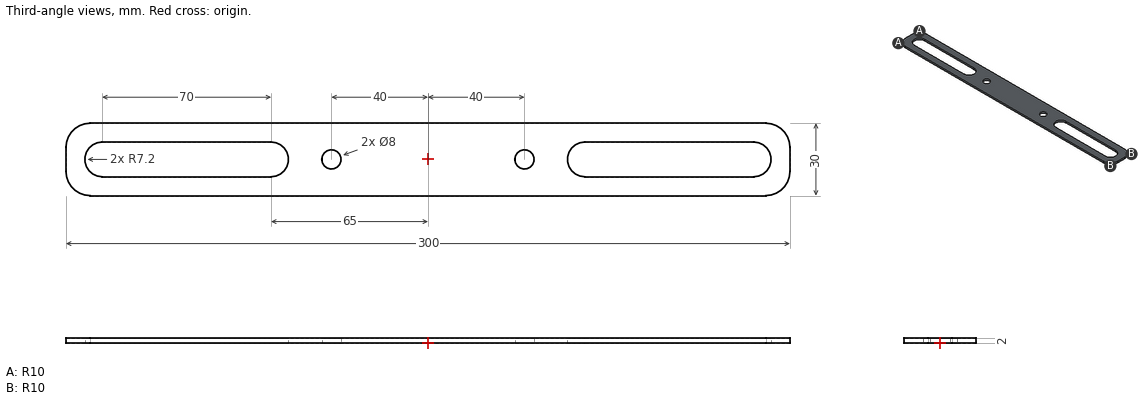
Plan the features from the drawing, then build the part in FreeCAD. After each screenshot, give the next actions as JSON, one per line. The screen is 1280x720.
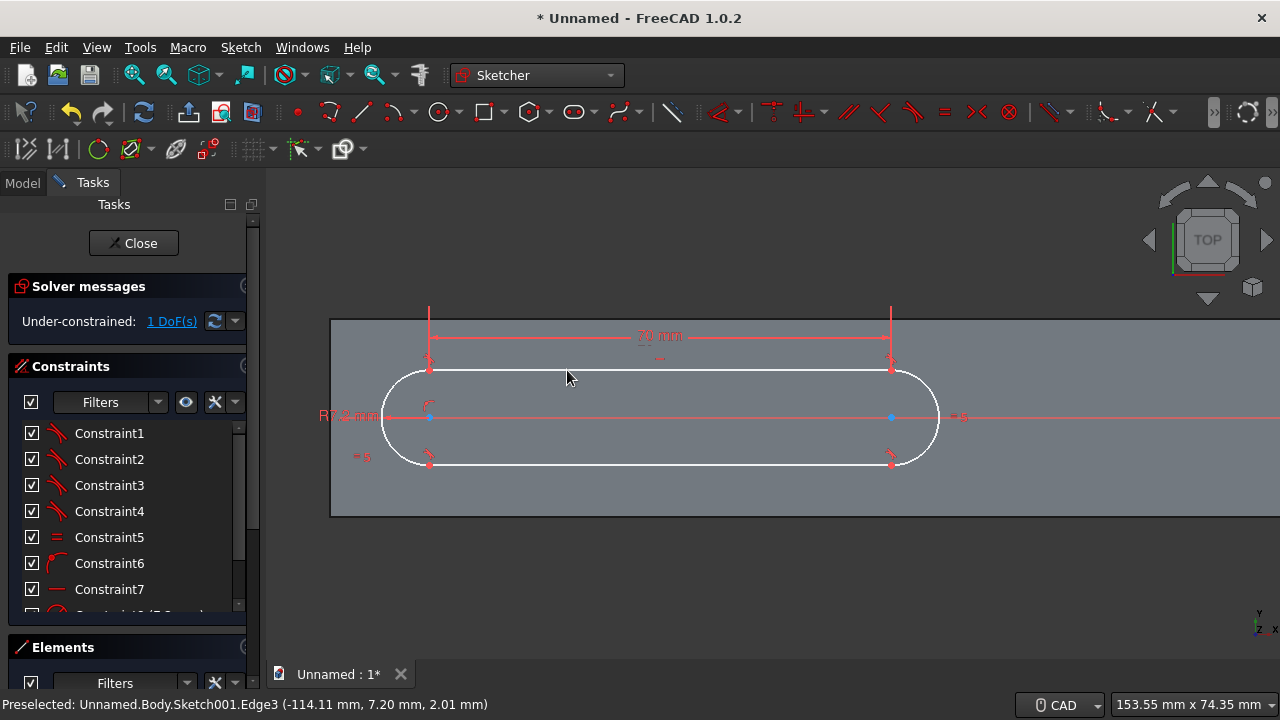
{"action": "left_click", "coordinate": [891, 465]}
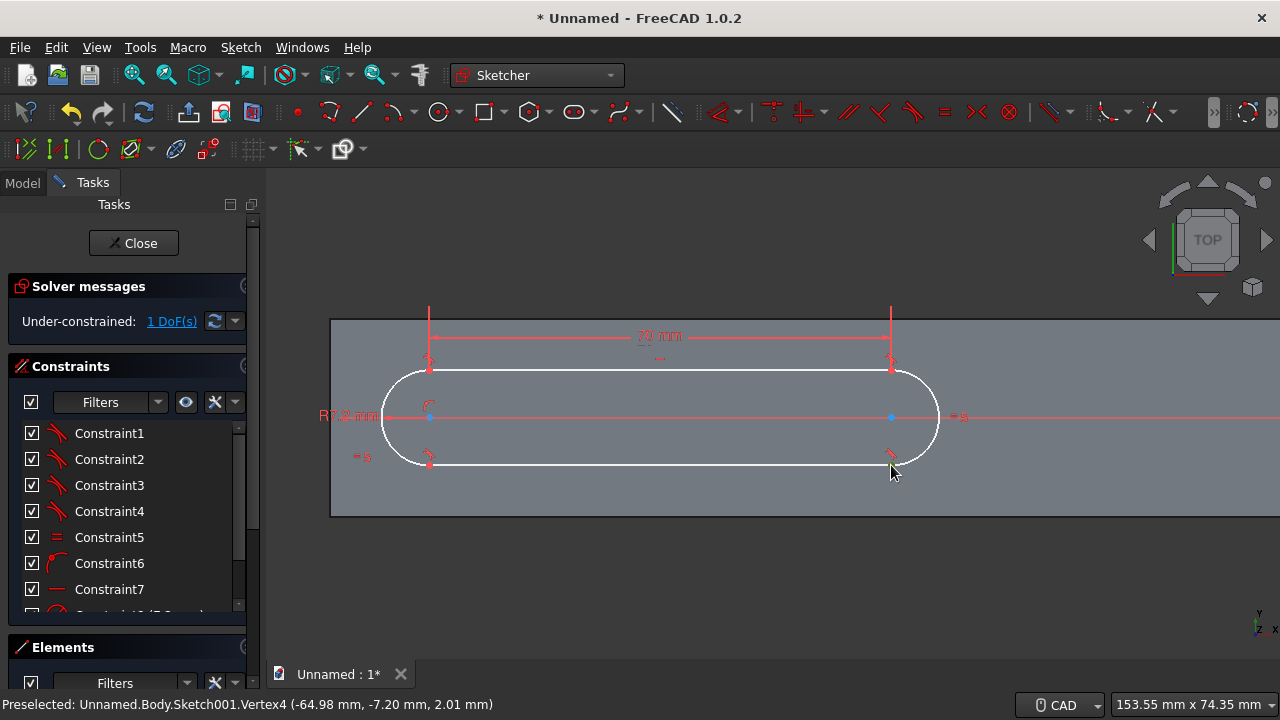
{"action": "key", "text": "l"}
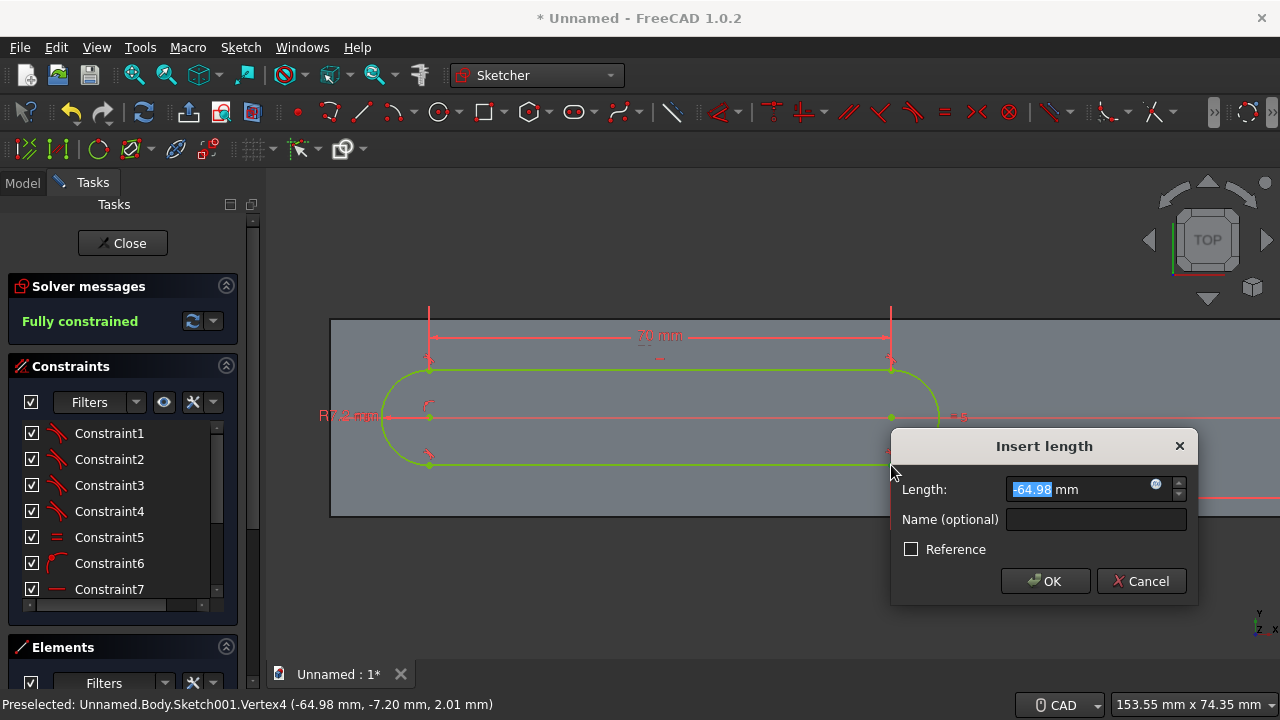
{"action": "type", "text": "-65"}
{"action": "key", "text": "Return"}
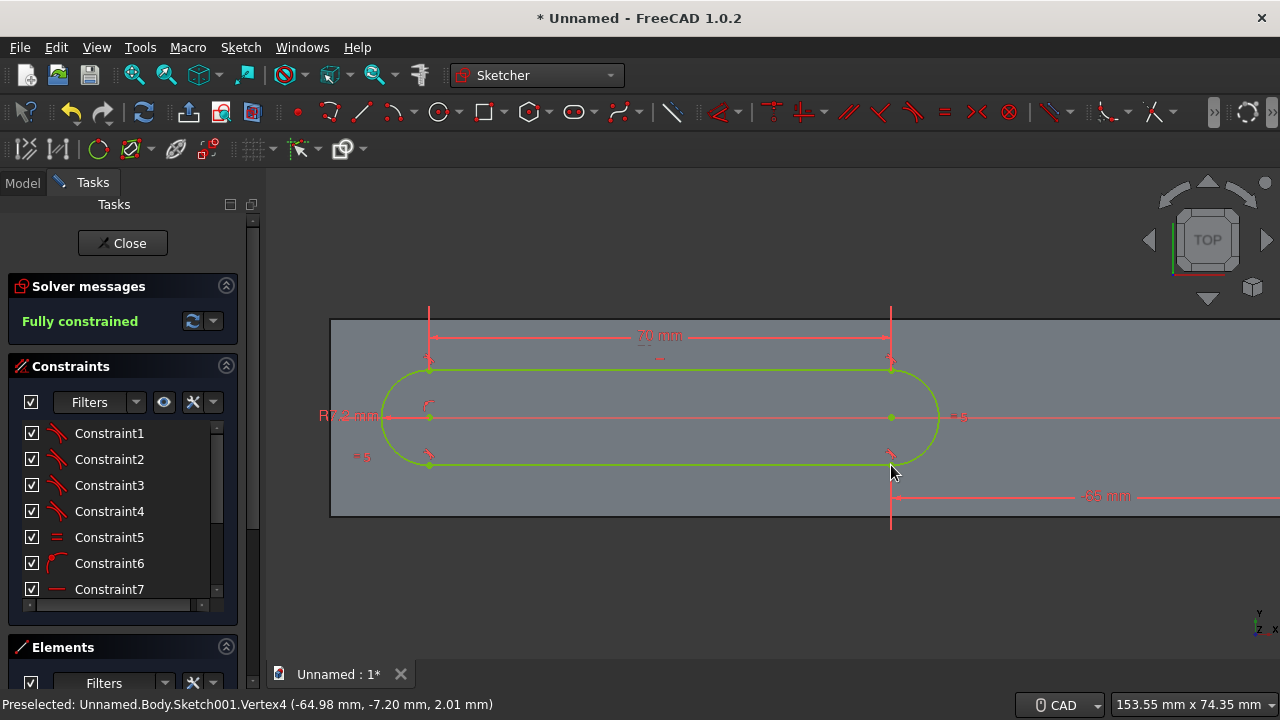
{"action": "left_click", "coordinate": [123, 243]}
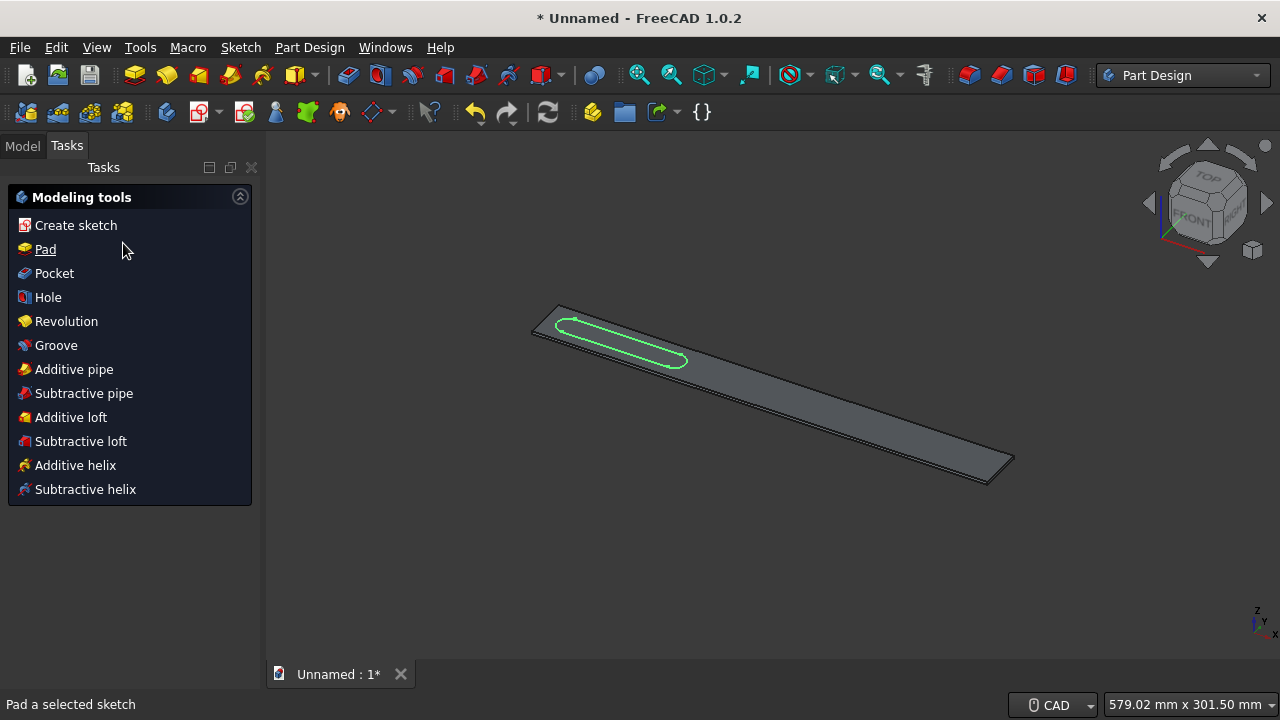
{"action": "left_click", "coordinate": [350, 76]}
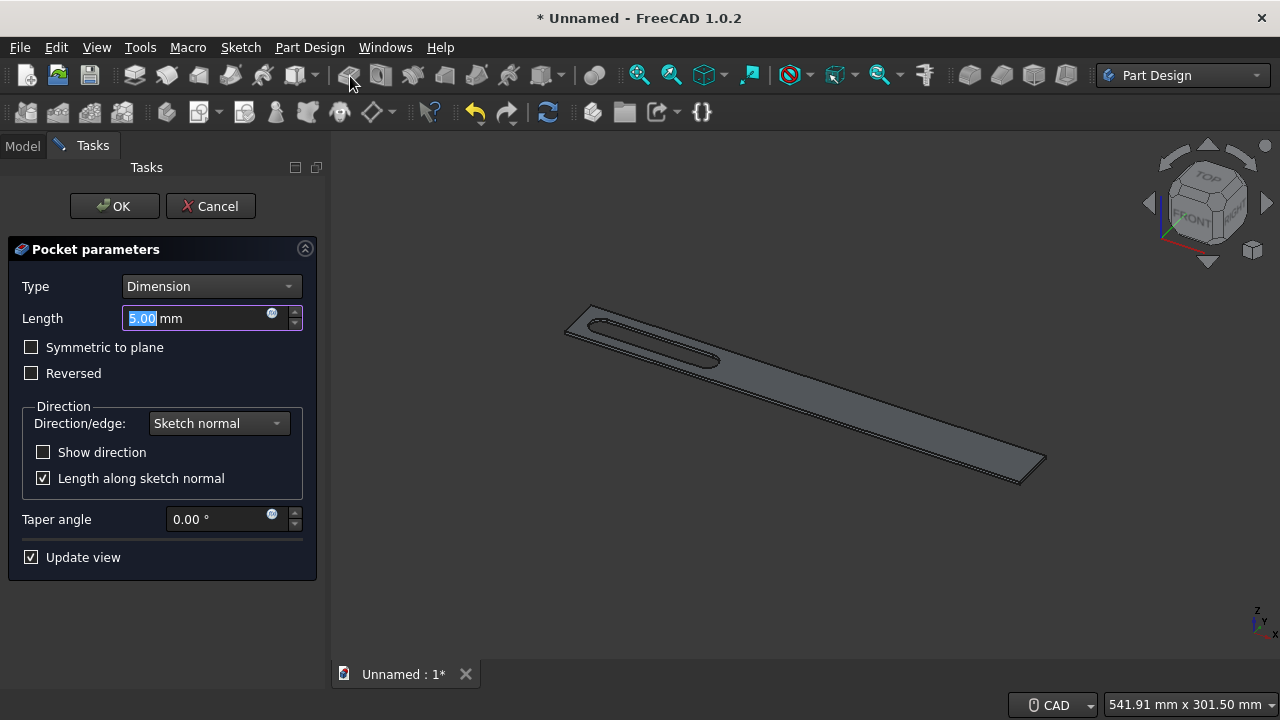
{"action": "left_click", "coordinate": [212, 286]}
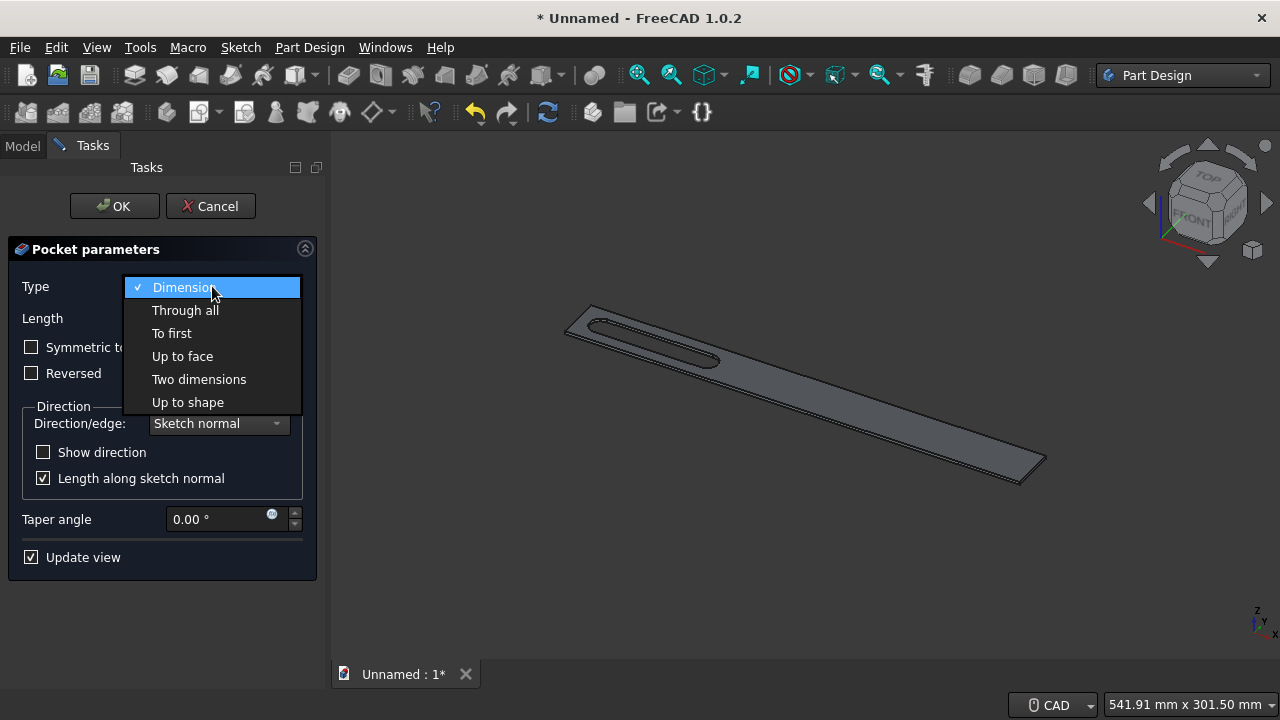
{"action": "left_click", "coordinate": [212, 310]}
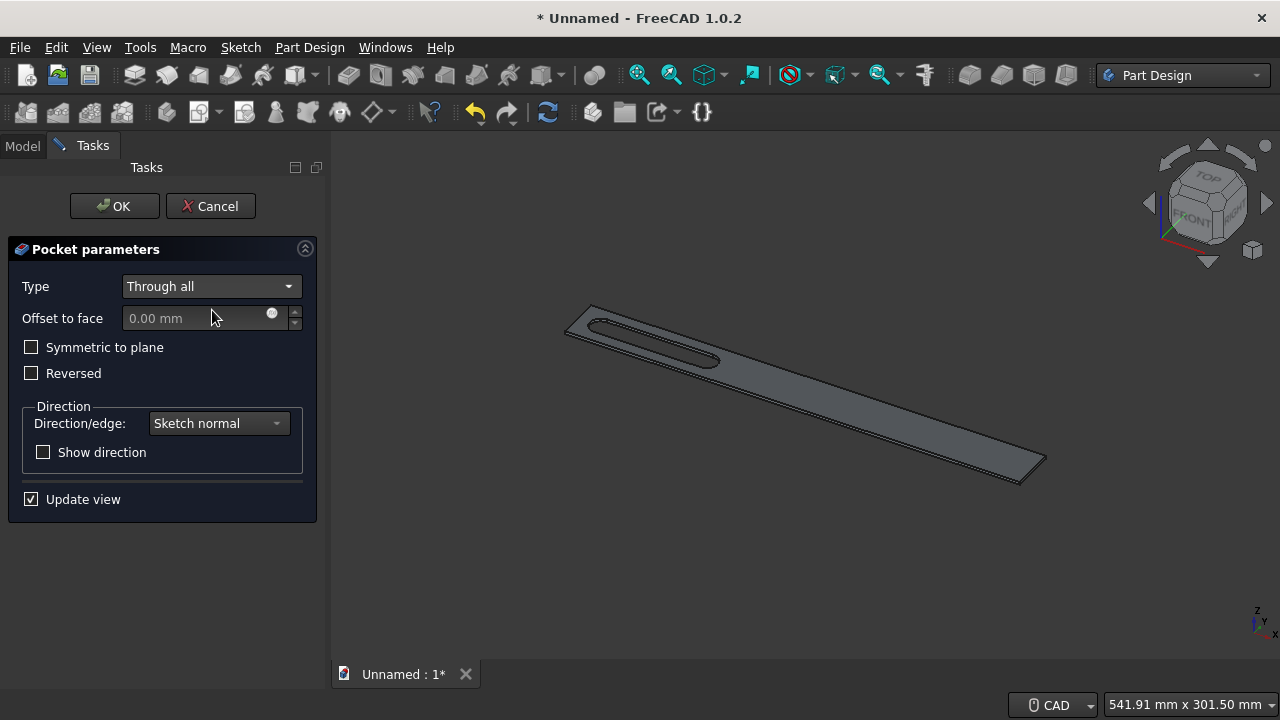
{"action": "left_click", "coordinate": [115, 206]}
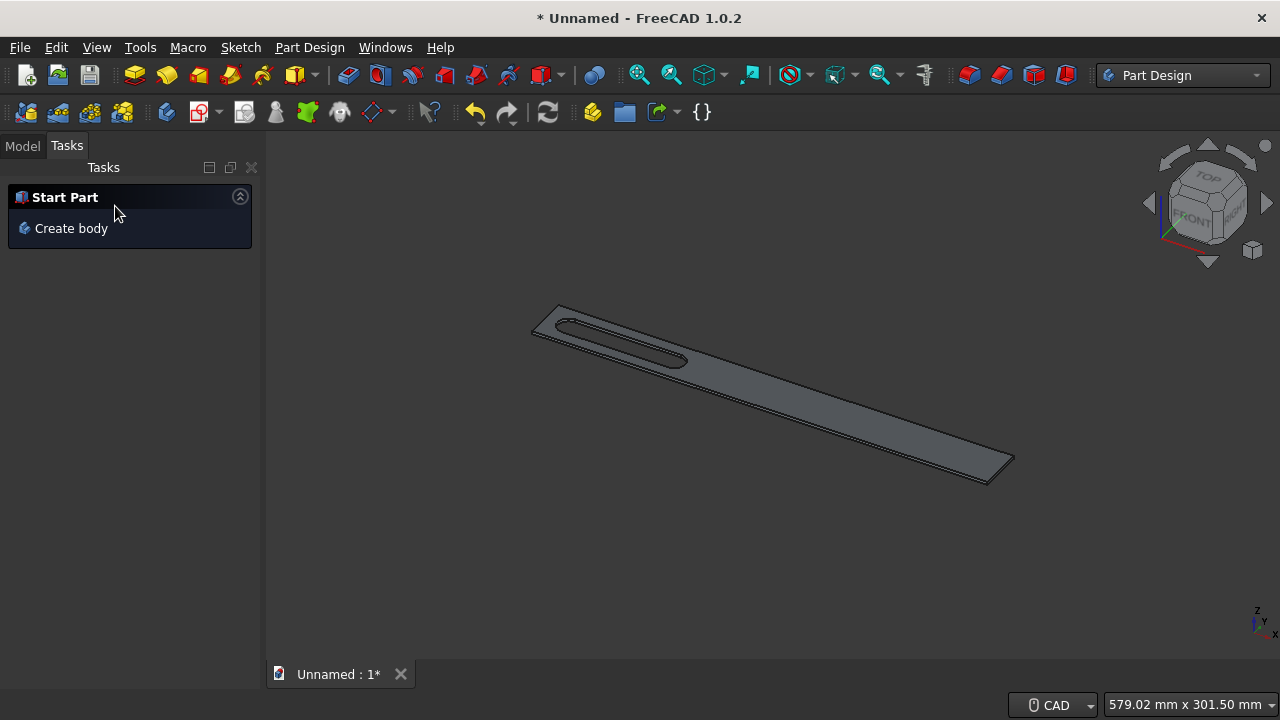
{"action": "scroll", "coordinate": [559, 306], "scroll_direction": "up", "scroll_amount": 13}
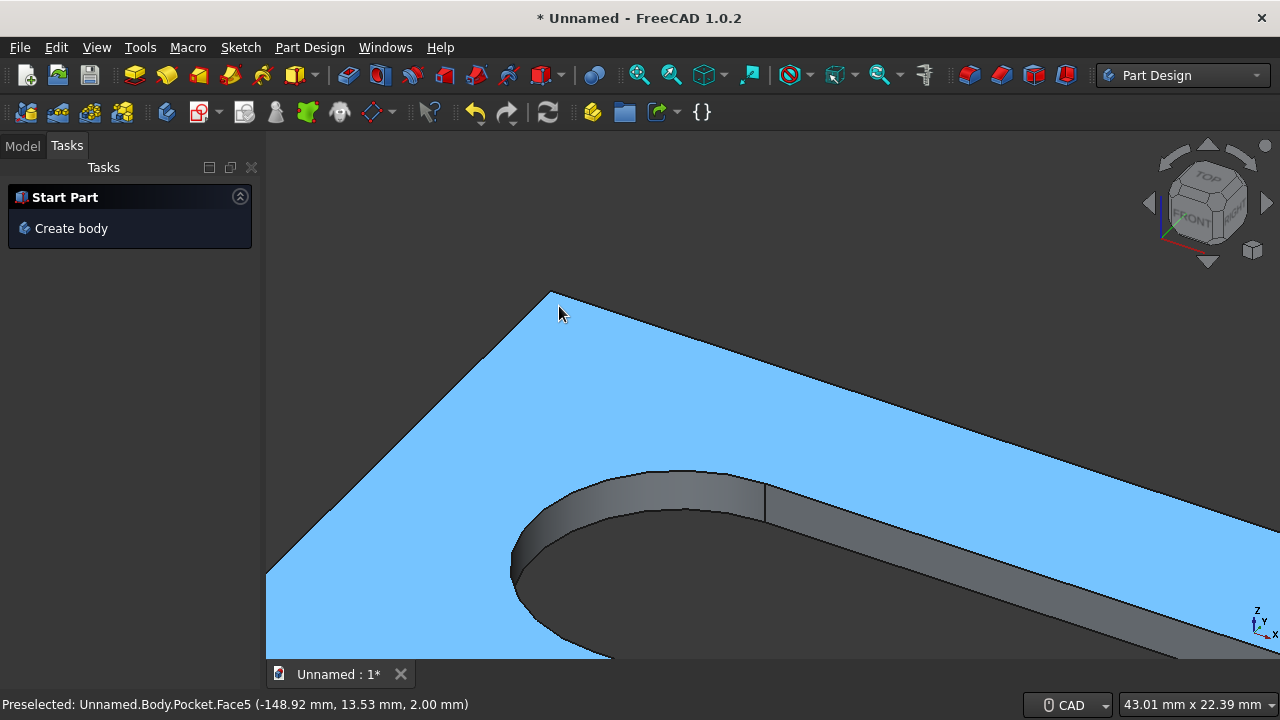
{"action": "key", "text": "v f"}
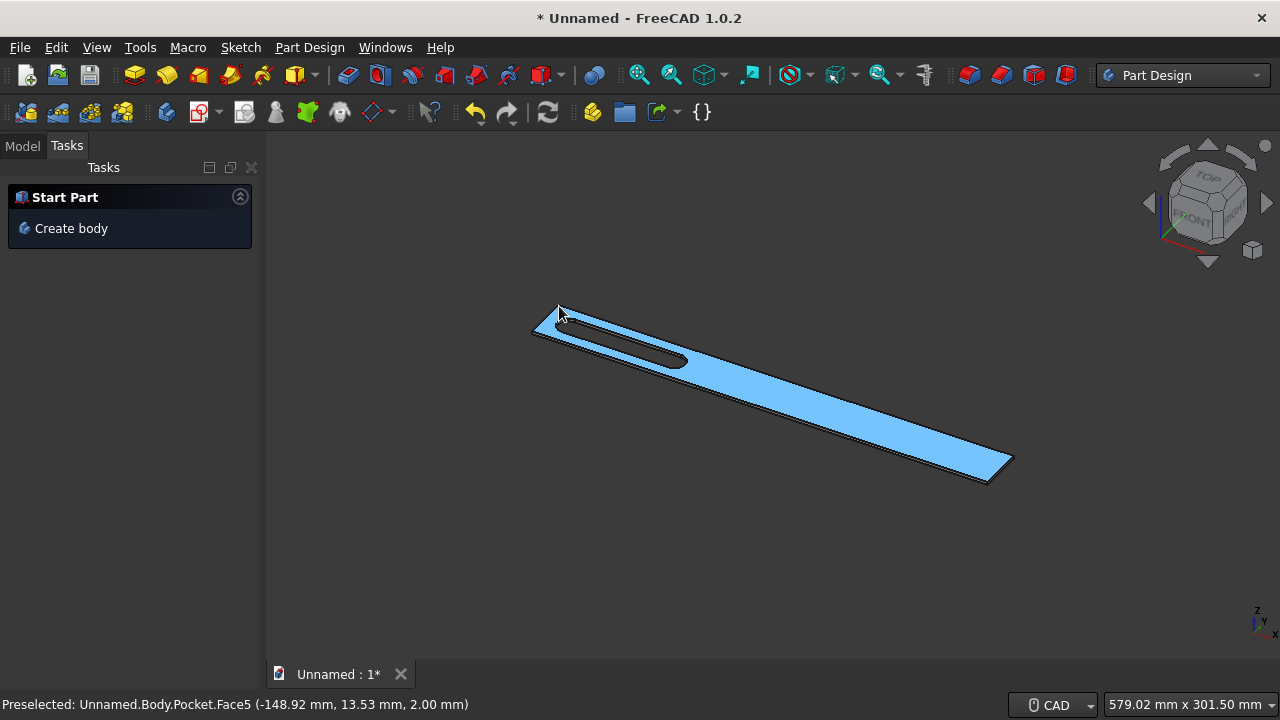
{"action": "key", "text": "0"}